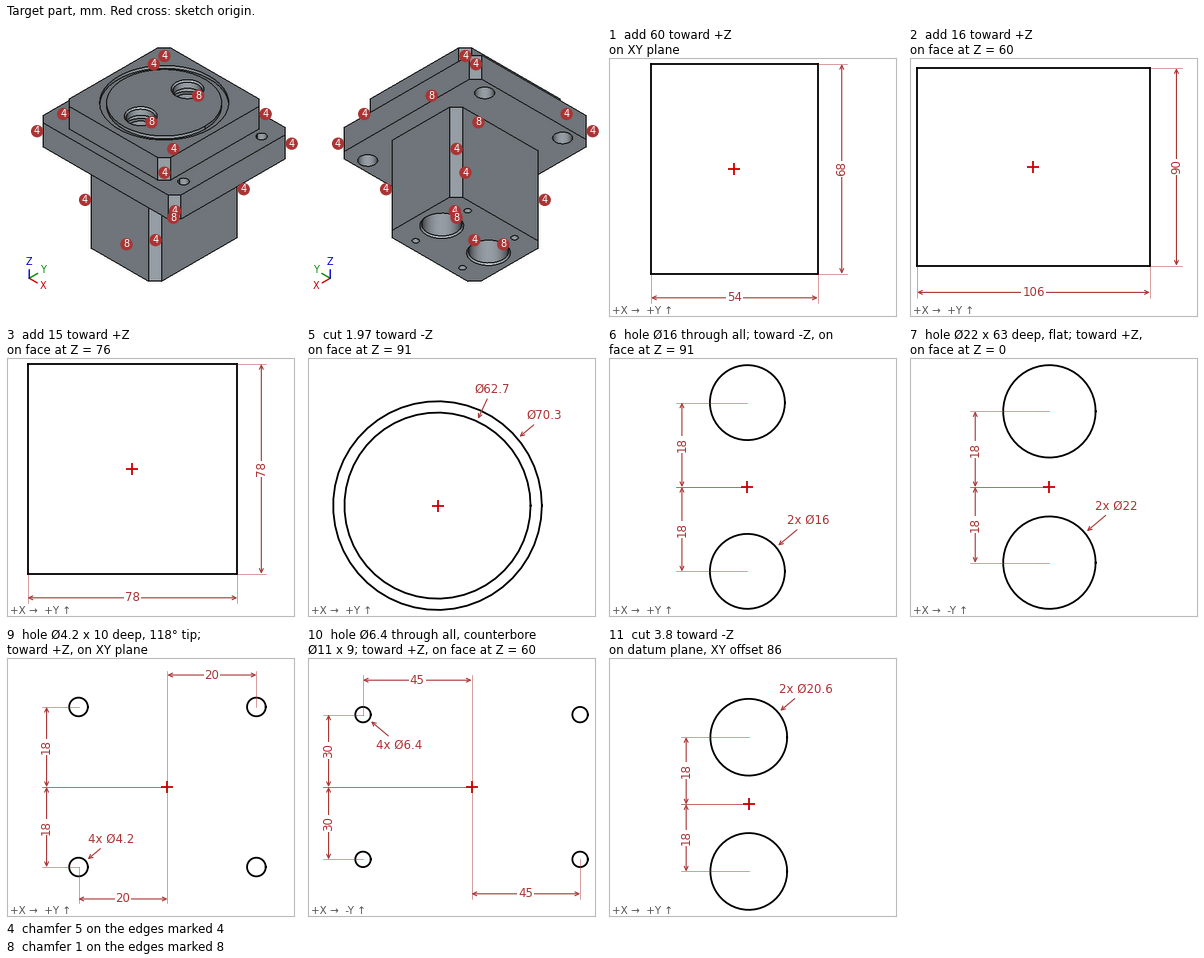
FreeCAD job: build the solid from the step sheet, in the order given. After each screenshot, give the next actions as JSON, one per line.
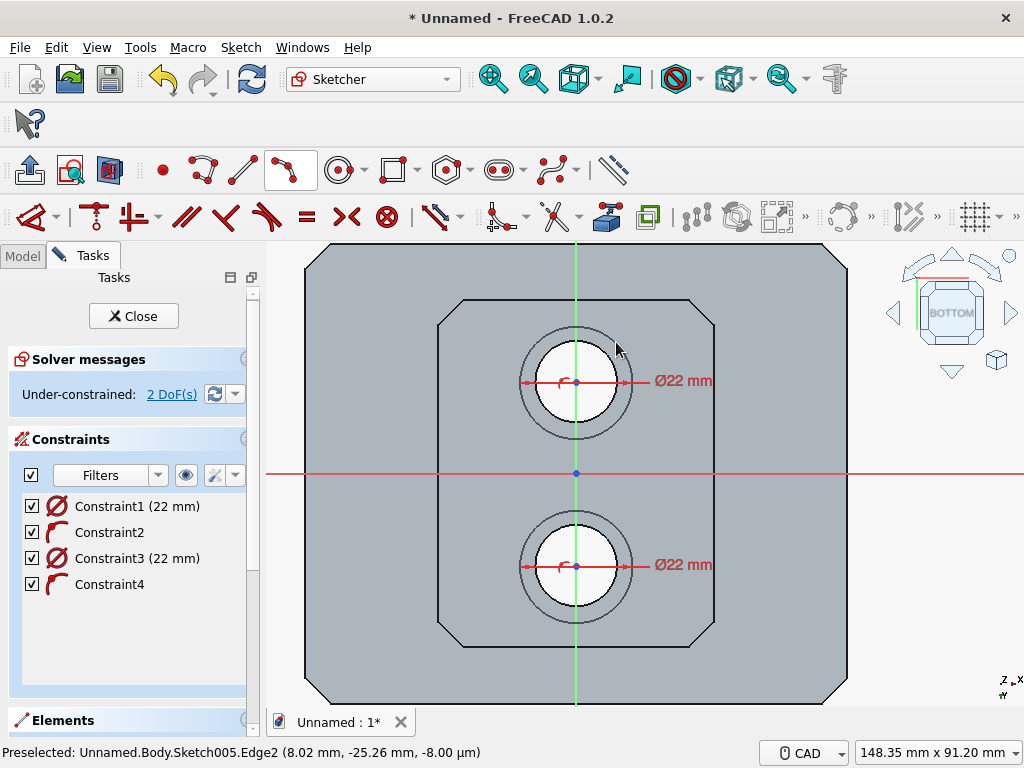
{"action": "key", "text": "d"}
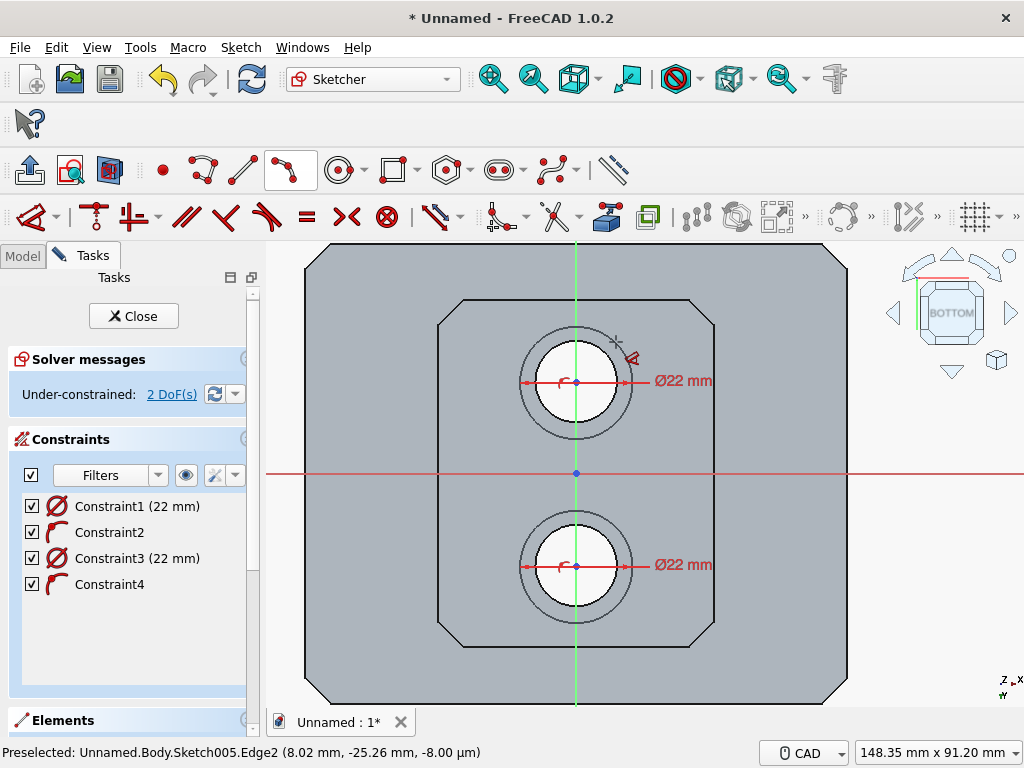
{"action": "left_click", "coordinate": [576, 567]}
{"action": "left_click", "coordinate": [610, 499]}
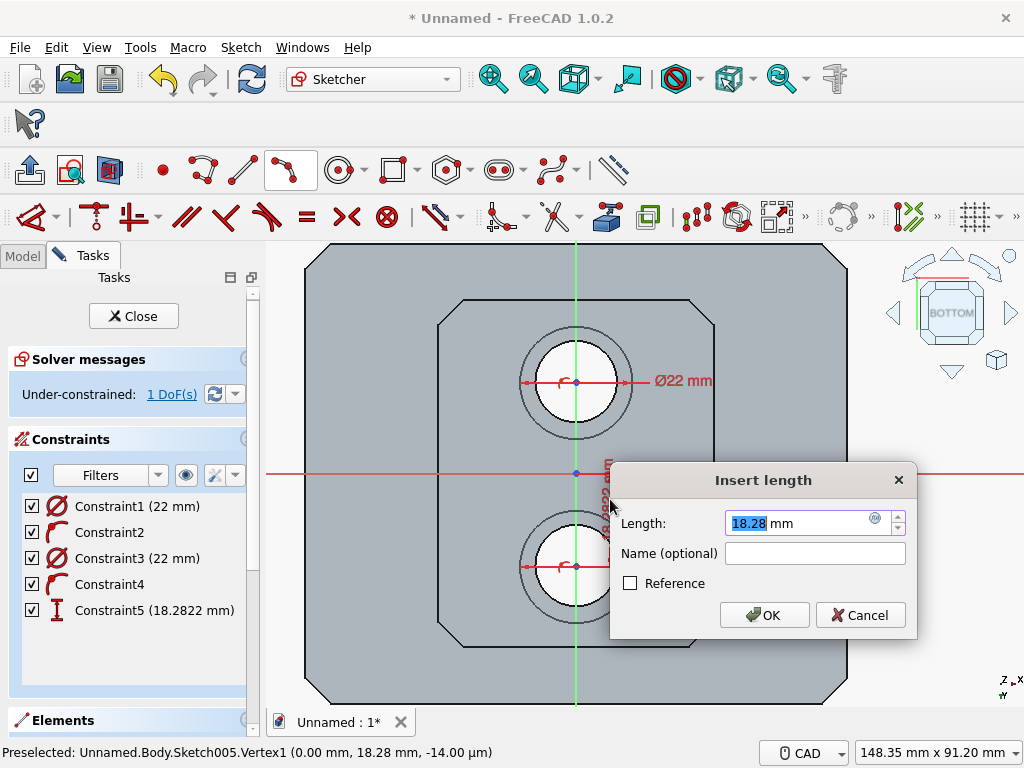
{"action": "type", "text": "18"}
{"action": "key", "text": "Return"}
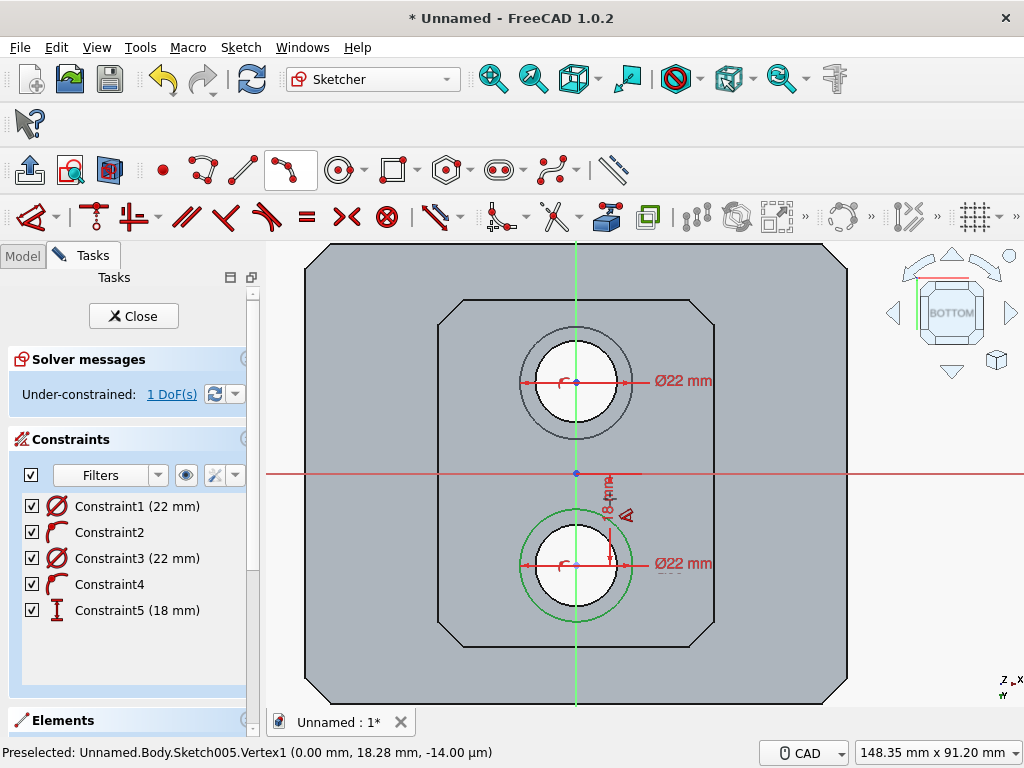
{"action": "left_click", "coordinate": [576, 383]}
{"action": "left_click", "coordinate": [610, 407]}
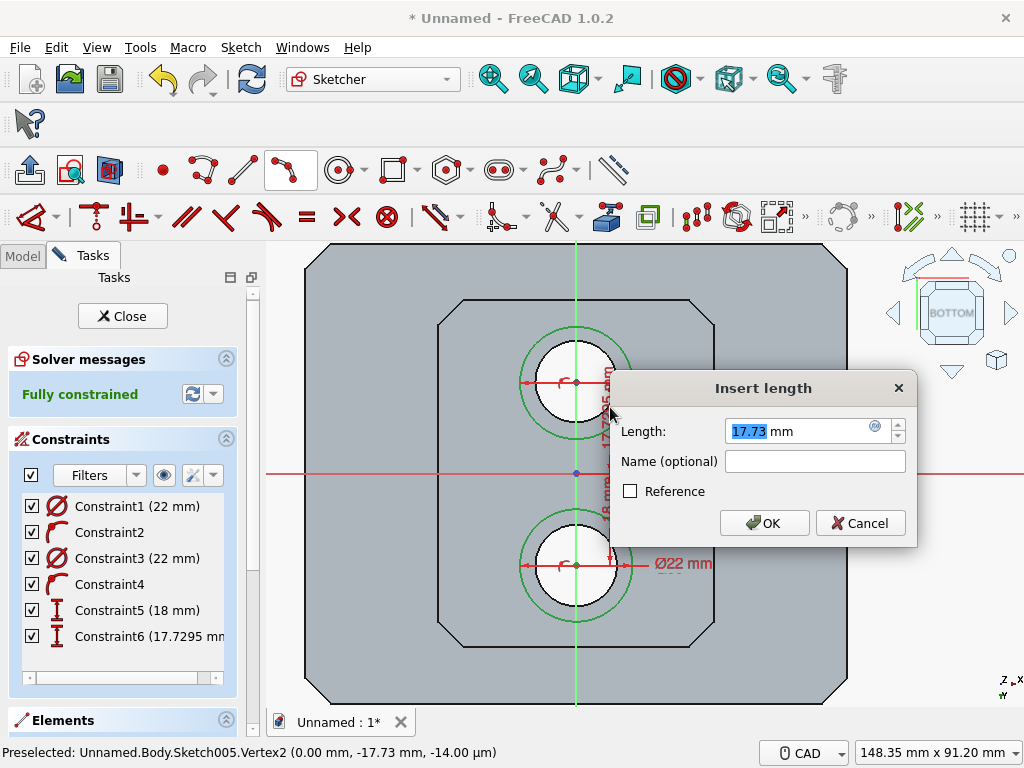
{"action": "type", "text": "18"}
{"action": "key", "text": "Return"}
{"action": "key", "text": "Escape"}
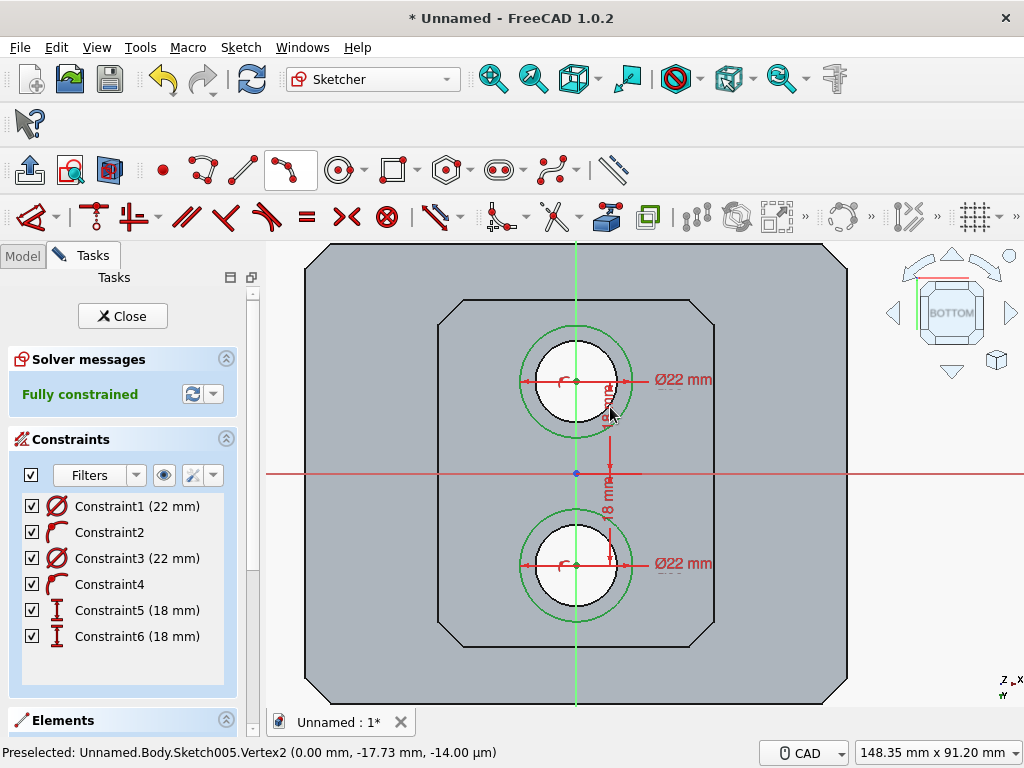
{"action": "left_click", "coordinate": [123, 316]}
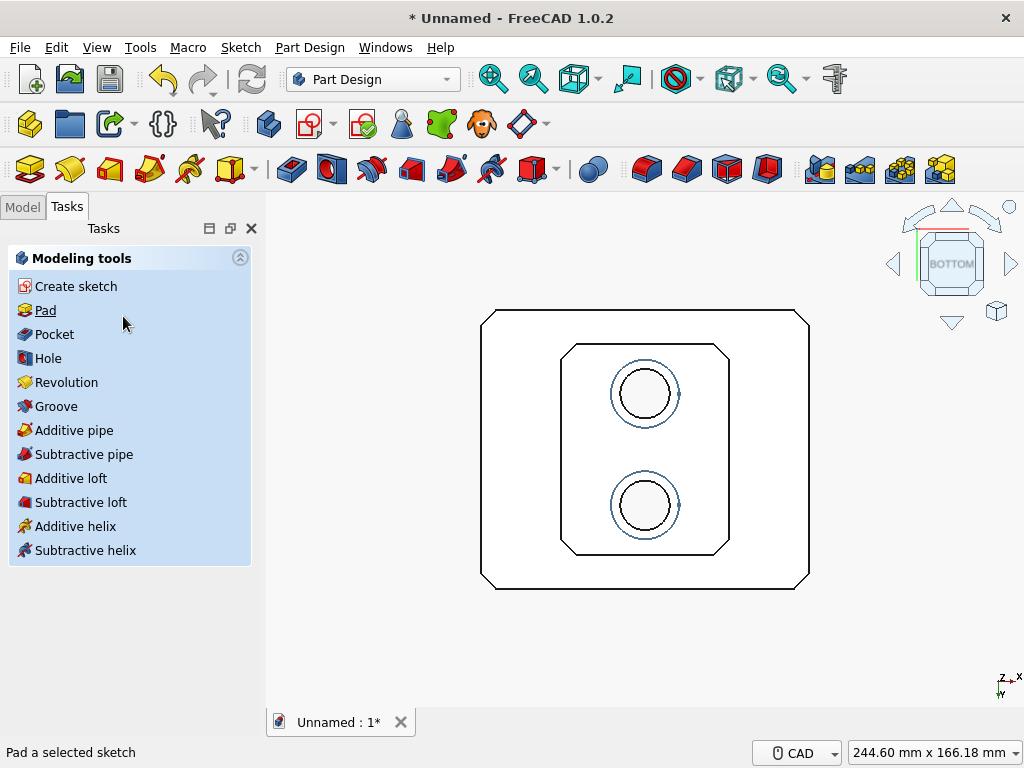
{"action": "left_click", "coordinate": [332, 170]}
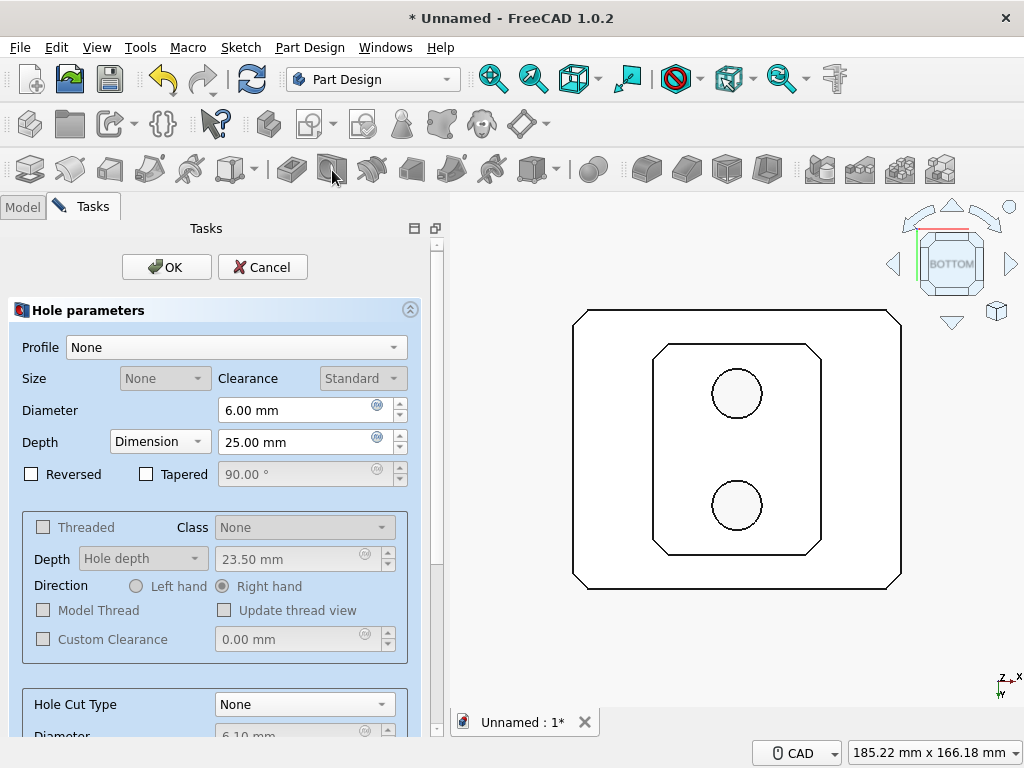
{"action": "triple_click", "coordinate": [305, 410]}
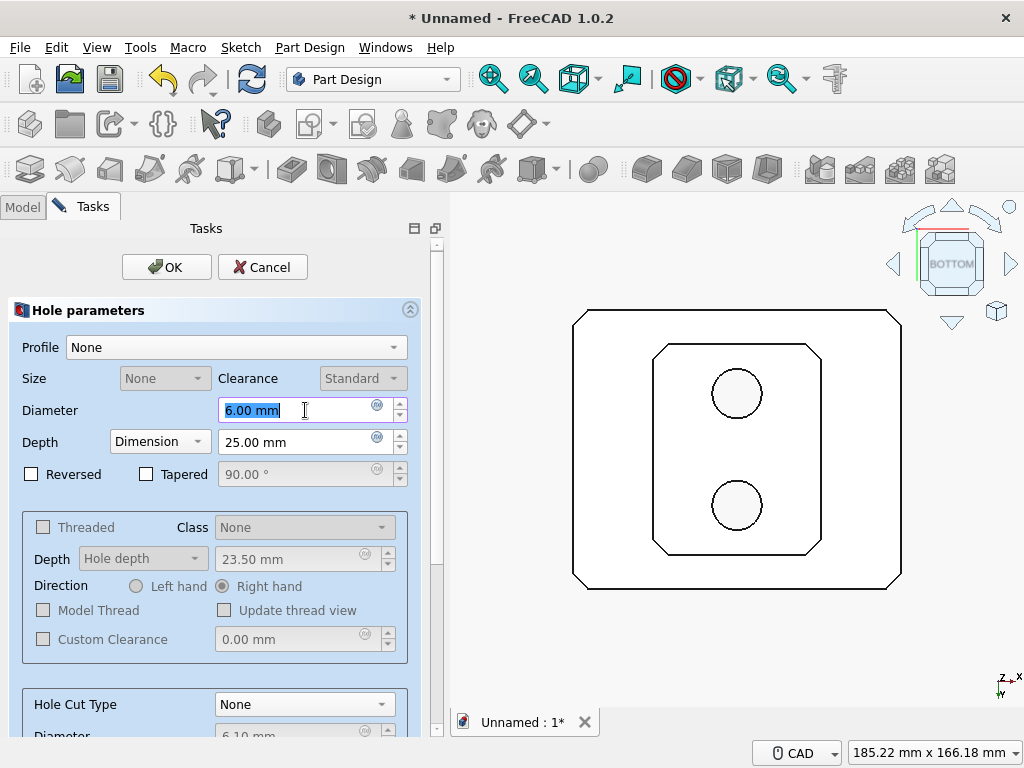
{"action": "type", "text": "22"}
{"action": "key", "text": "Tab"}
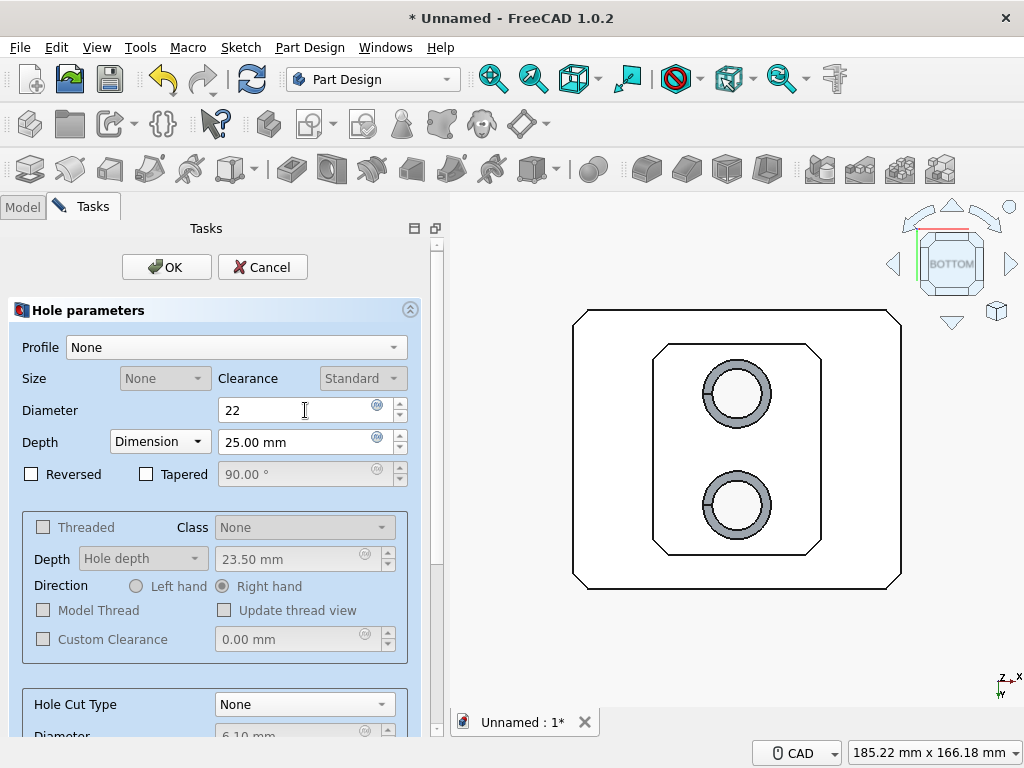
{"action": "triple_click", "coordinate": [305, 442]}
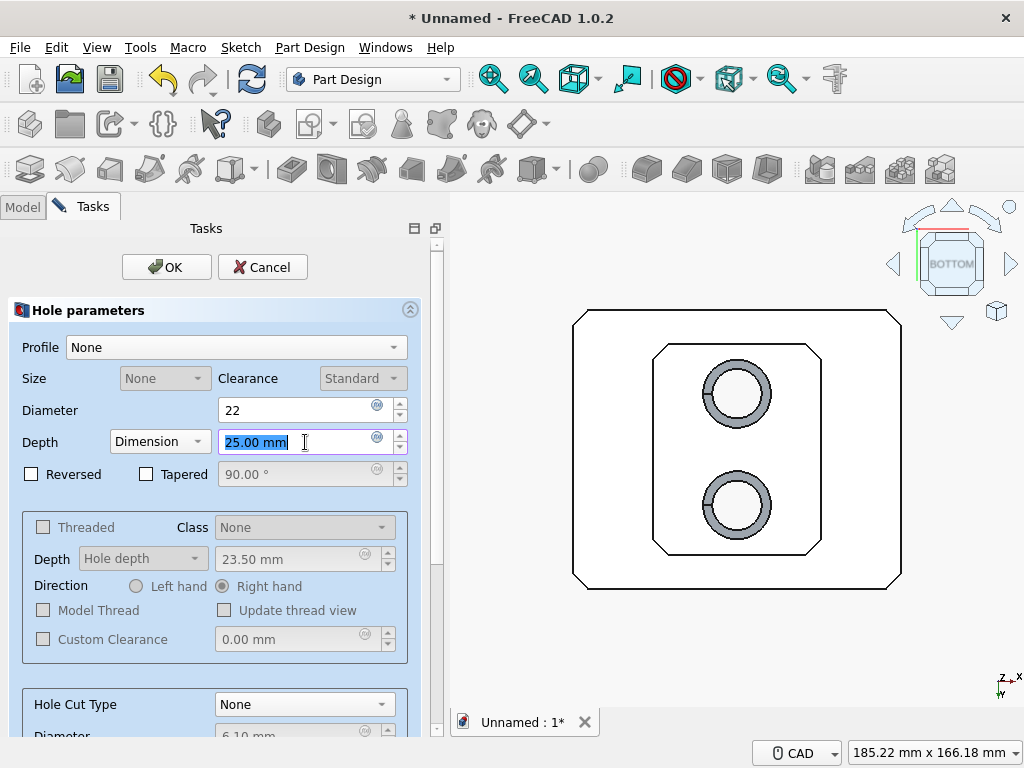
{"action": "type", "text": "63"}
{"action": "key", "text": "Tab"}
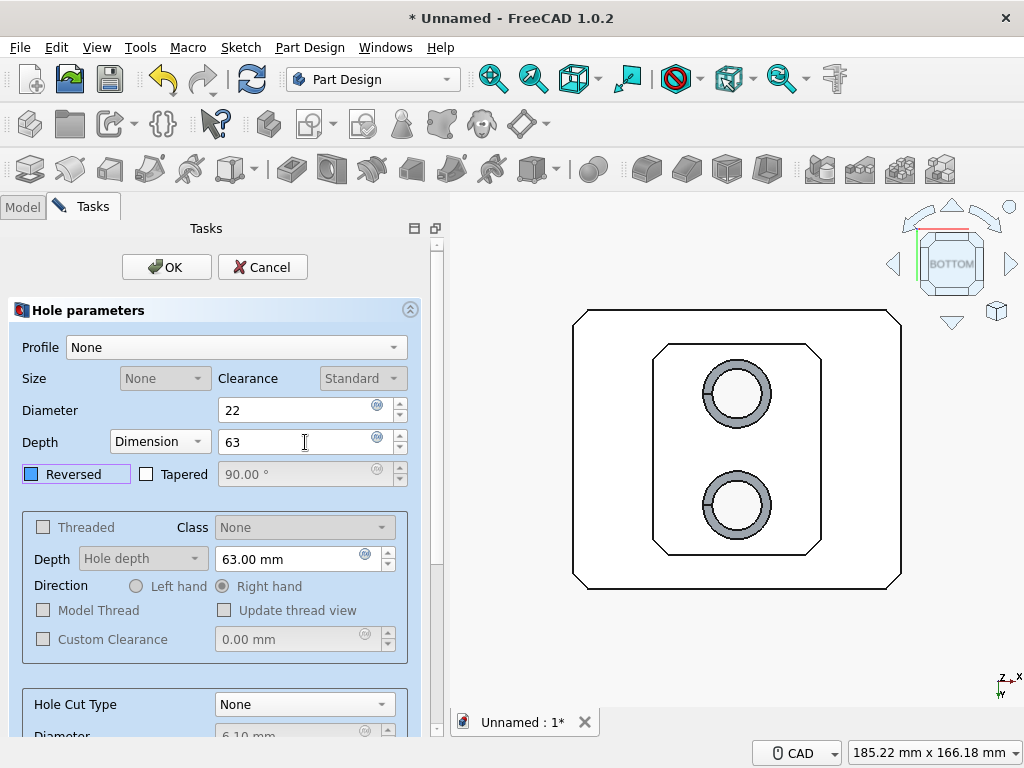
{"action": "scroll", "coordinate": [437, 487], "scroll_direction": "down", "scroll_amount": 4}